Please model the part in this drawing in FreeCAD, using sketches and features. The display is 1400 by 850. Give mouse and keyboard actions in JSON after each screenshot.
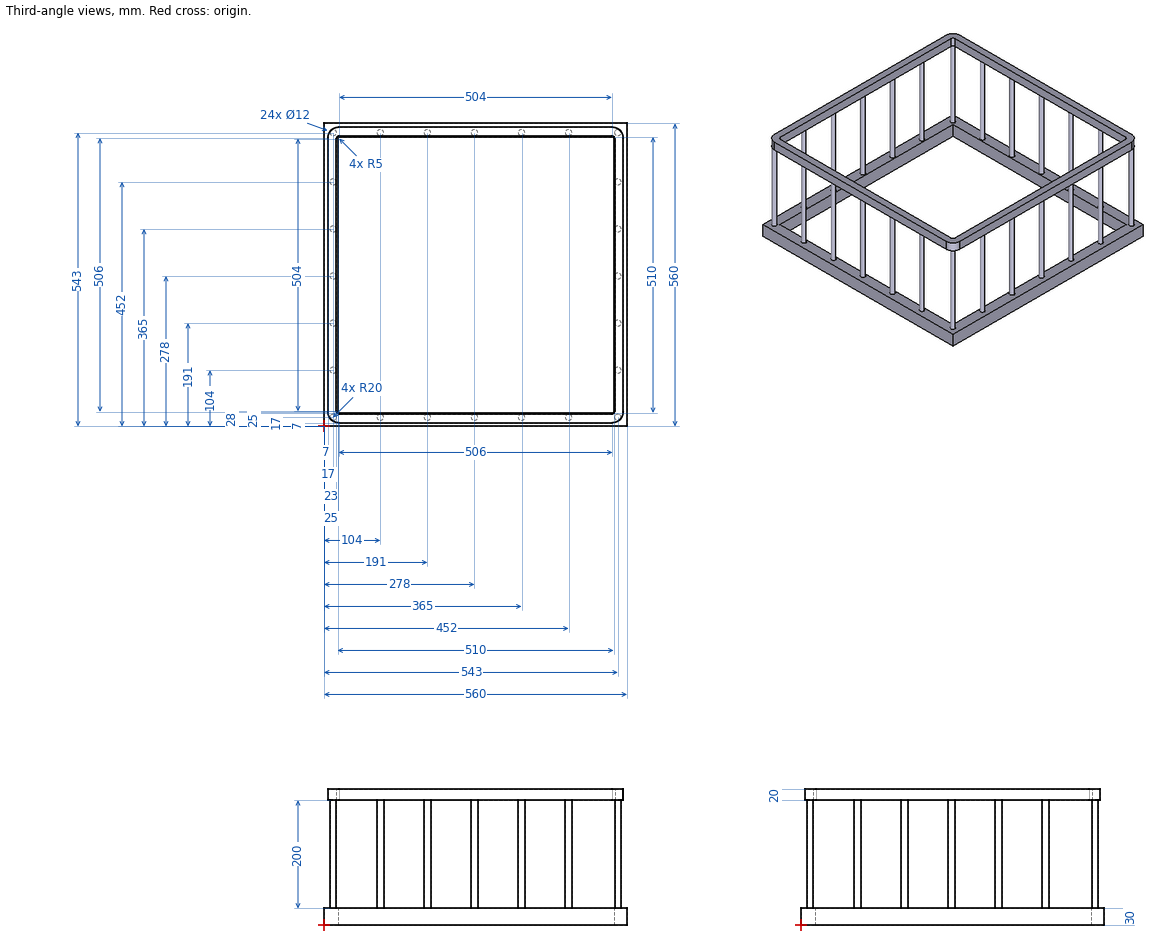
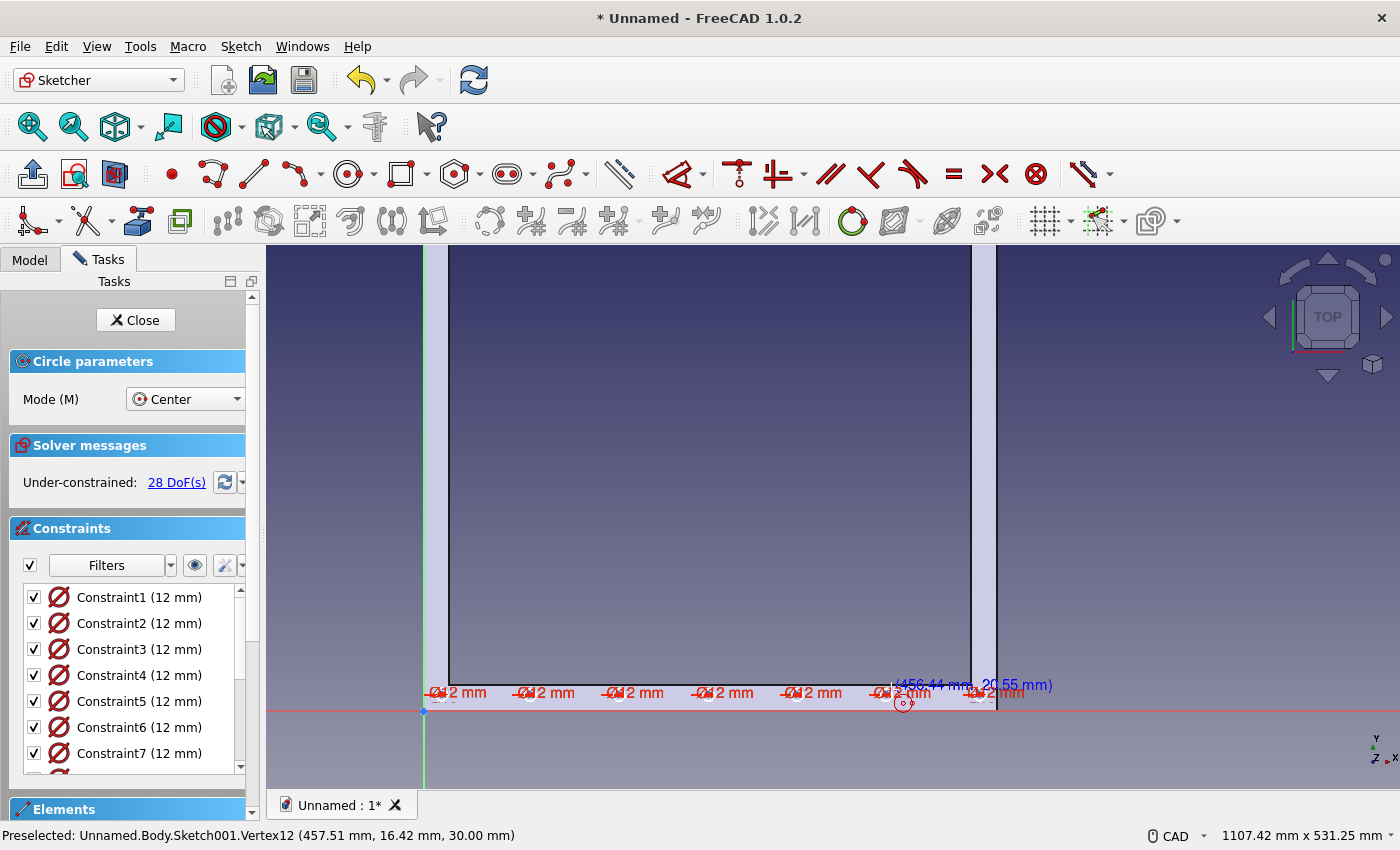
{"action": "scroll", "coordinate": [441, 605], "scroll_direction": "up", "scroll_amount": 7}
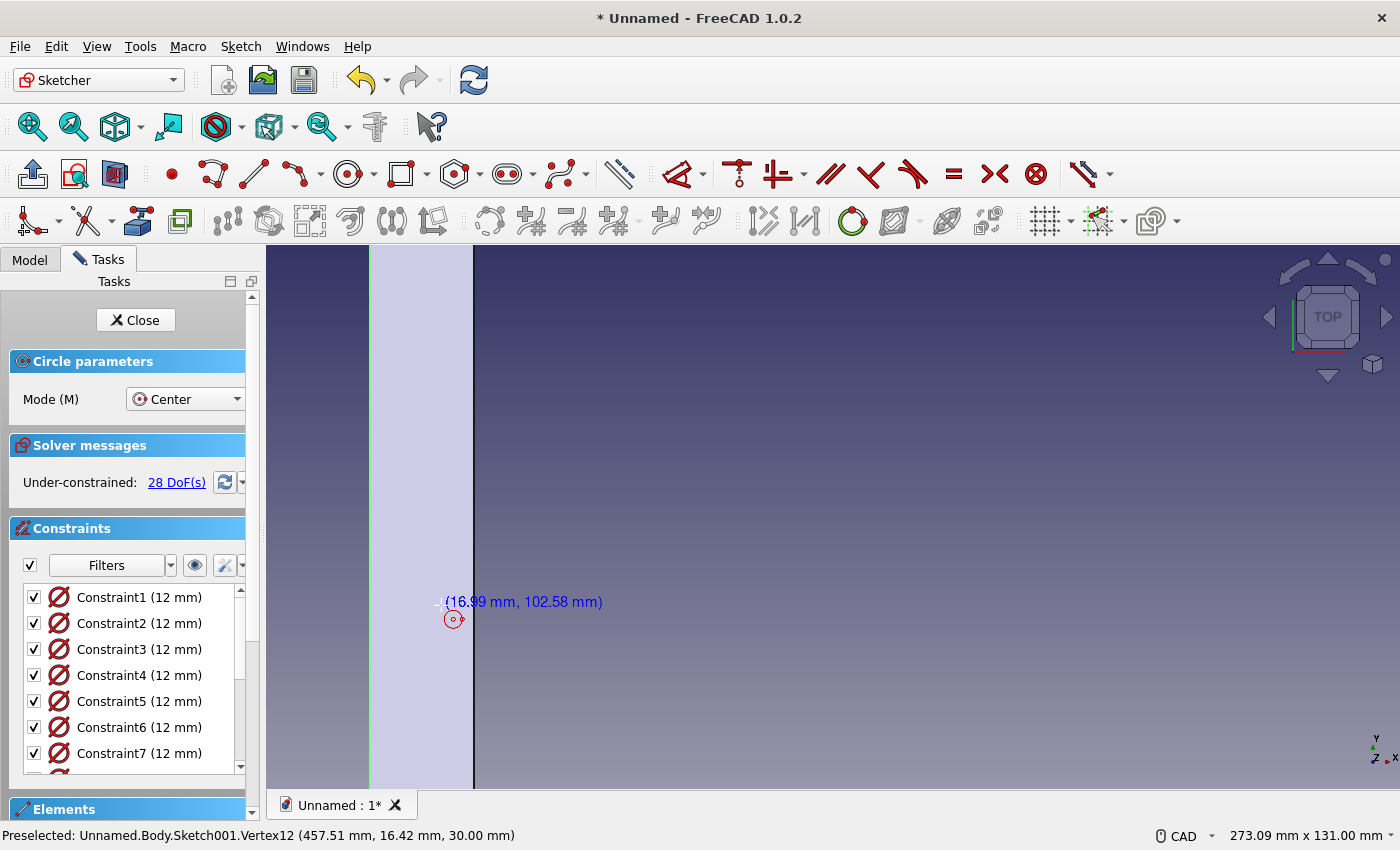
{"action": "scroll", "coordinate": [617, 641], "scroll_direction": "down", "scroll_amount": 9}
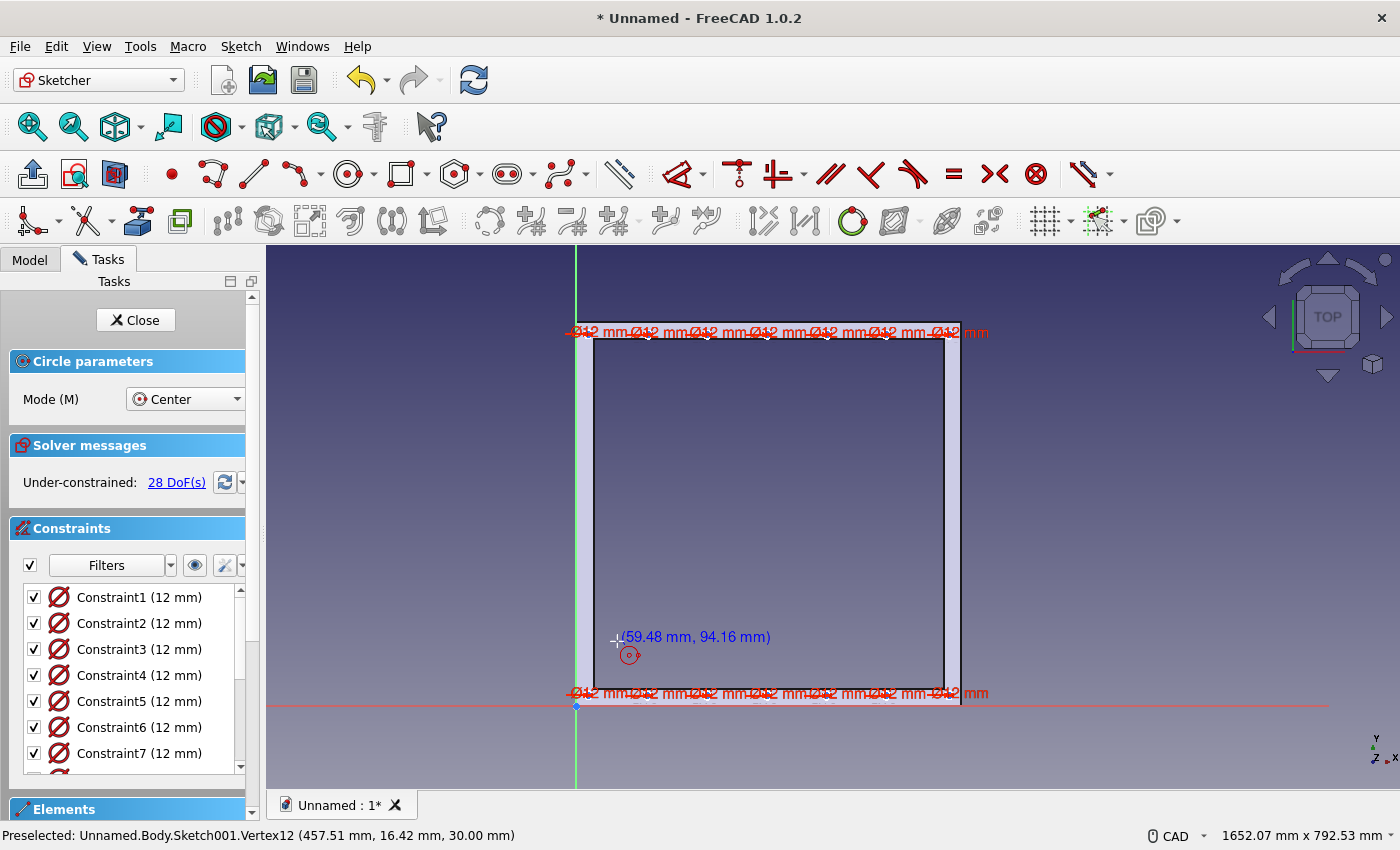
{"action": "scroll", "coordinate": [588, 635], "scroll_direction": "up", "scroll_amount": 2}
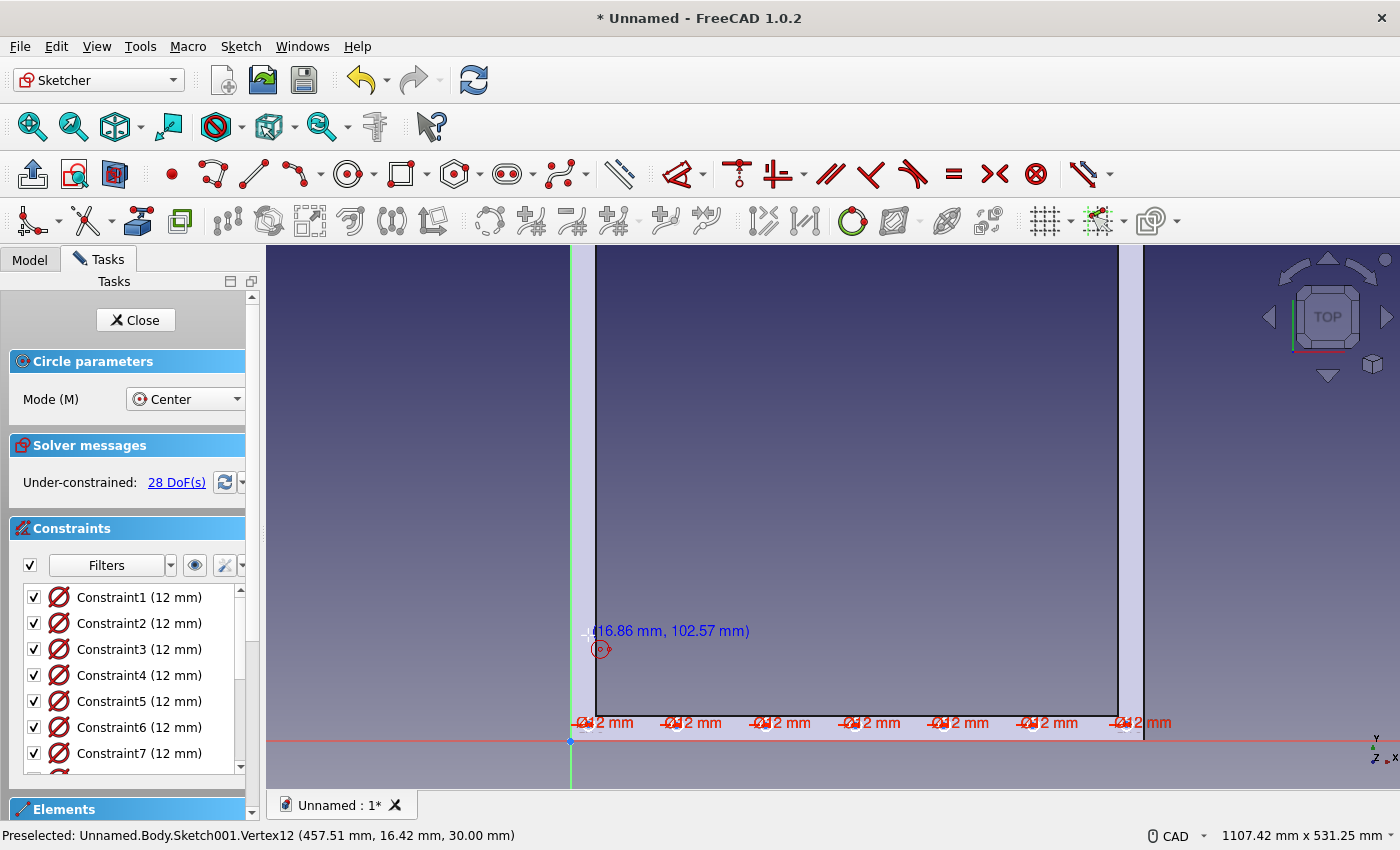
{"action": "left_click", "coordinate": [588, 635]}
{"action": "mouse_move", "coordinate": [592, 630]}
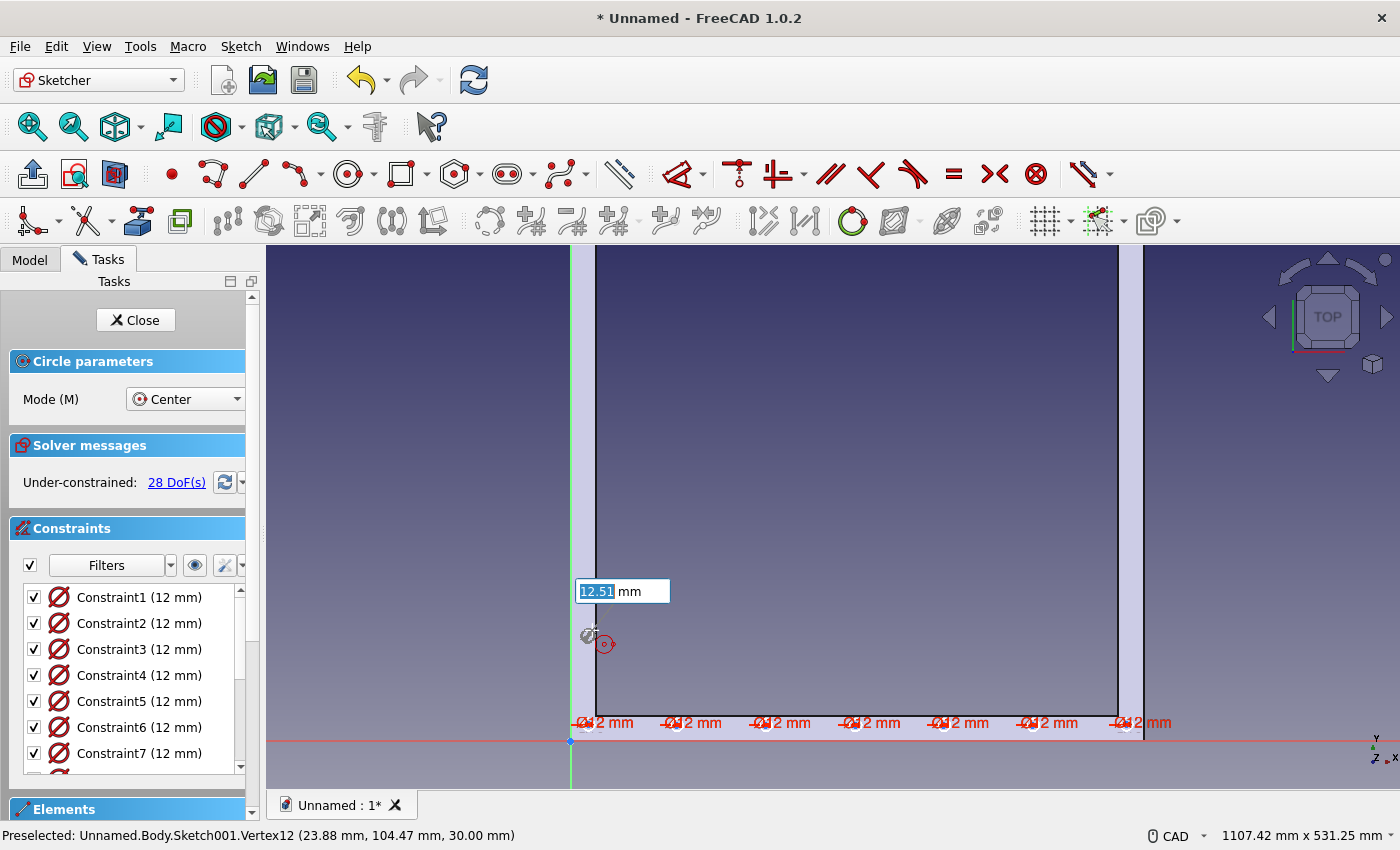
{"action": "type", "text": "12"}
{"action": "key", "text": "Return"}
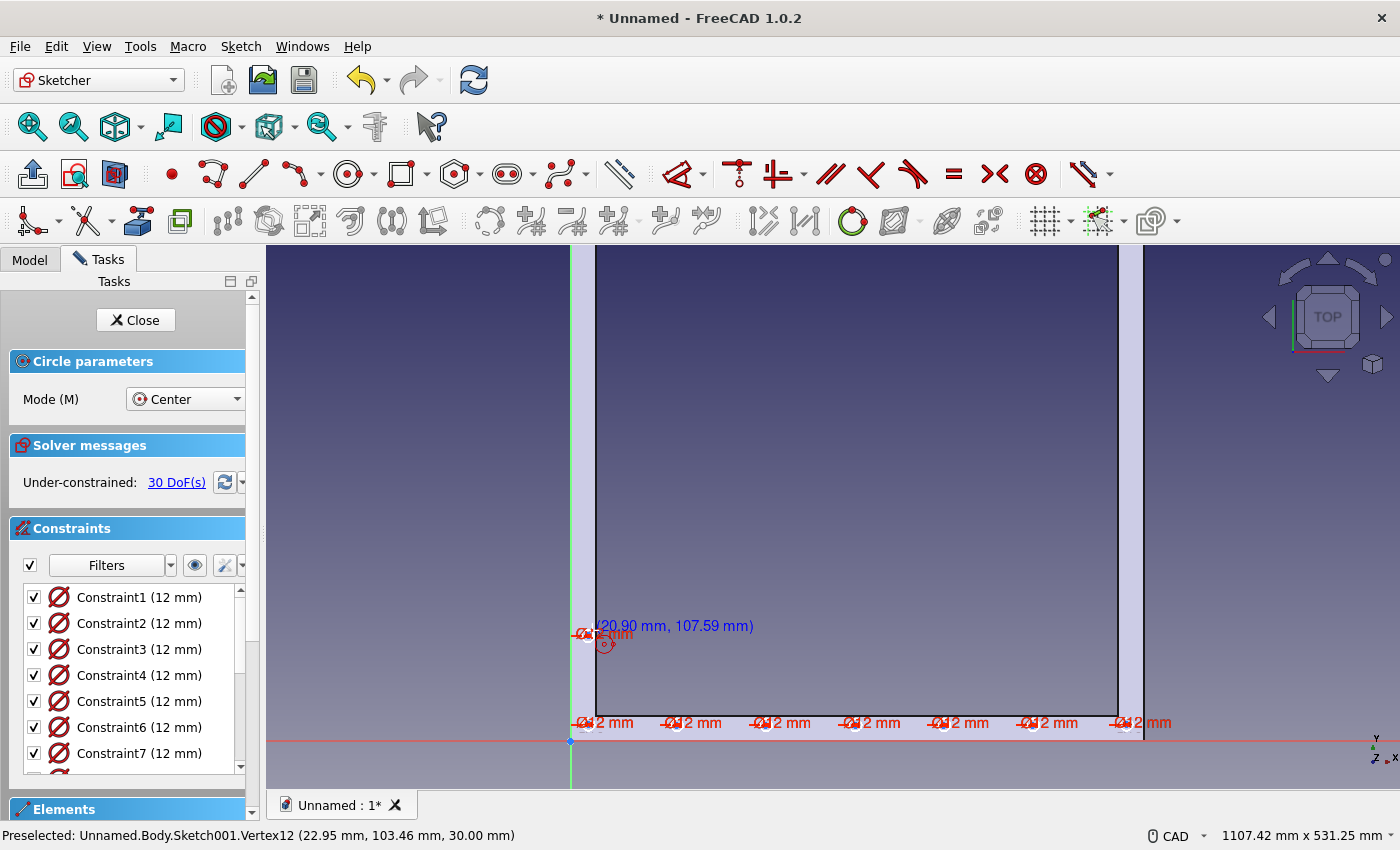
{"action": "scroll", "coordinate": [1127, 635], "scroll_direction": "up", "scroll_amount": 7}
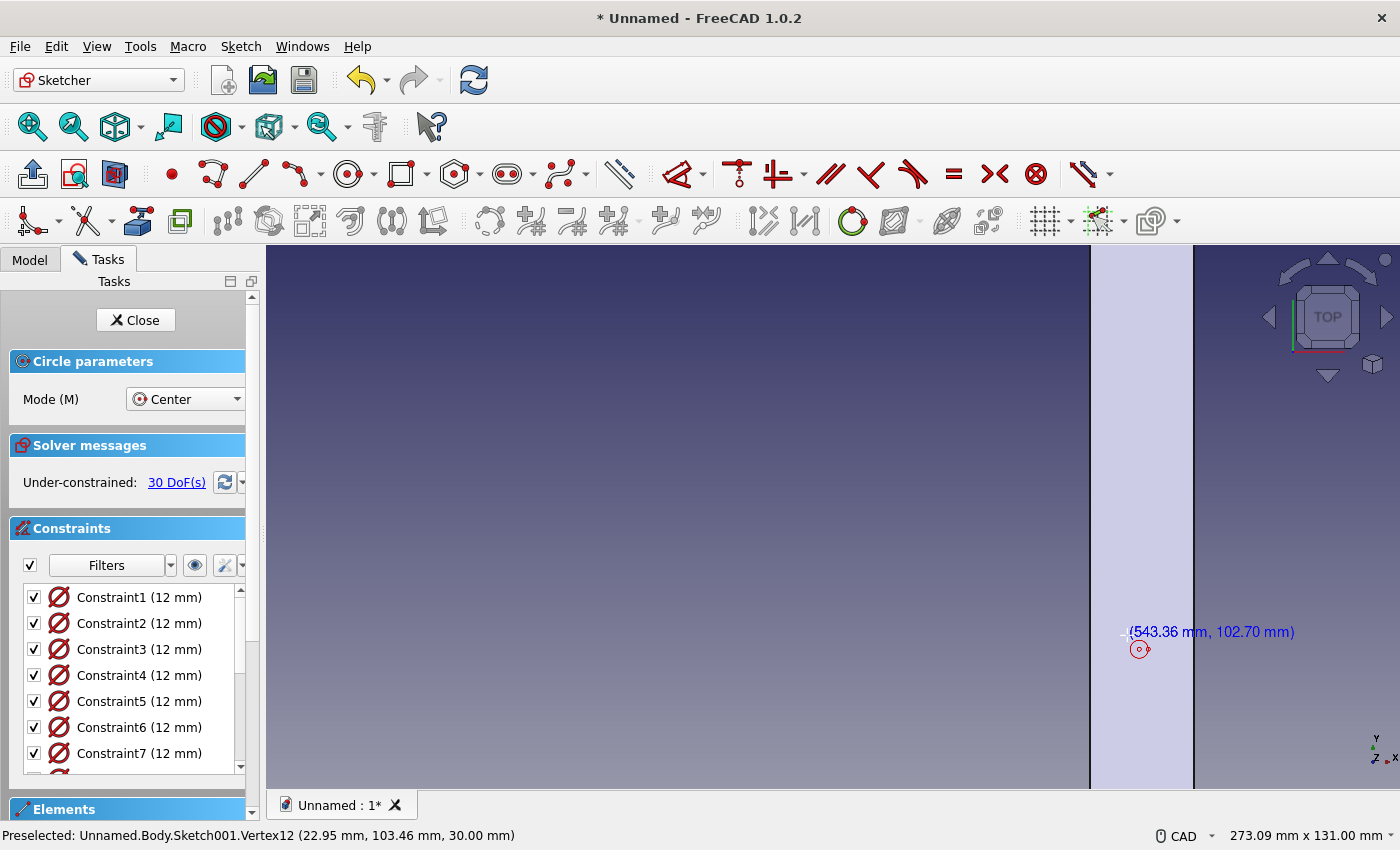
{"action": "scroll", "coordinate": [914, 635], "scroll_direction": "down", "scroll_amount": 9}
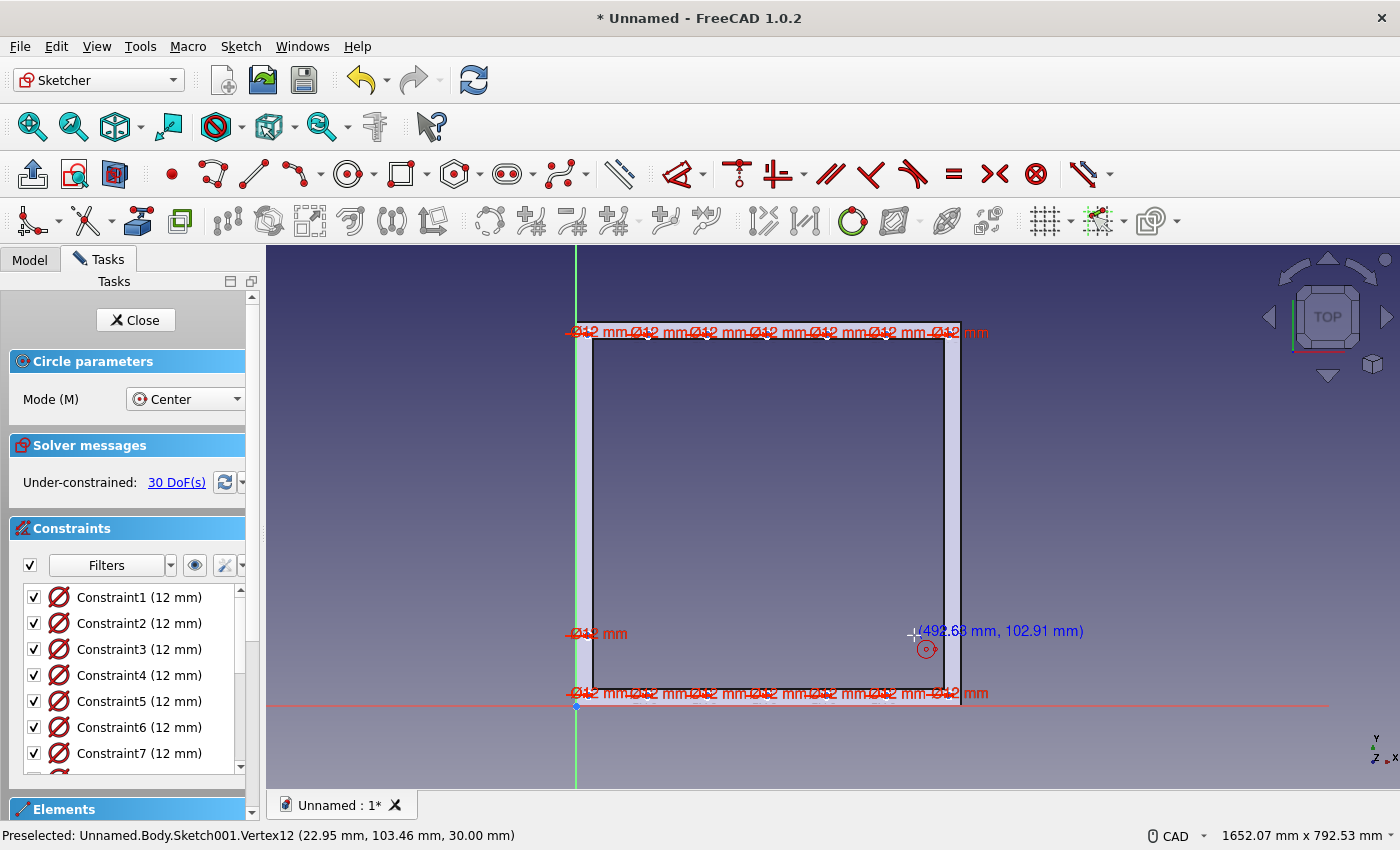
{"action": "left_click", "coordinate": [949, 635]}
{"action": "mouse_move", "coordinate": [952, 632]}